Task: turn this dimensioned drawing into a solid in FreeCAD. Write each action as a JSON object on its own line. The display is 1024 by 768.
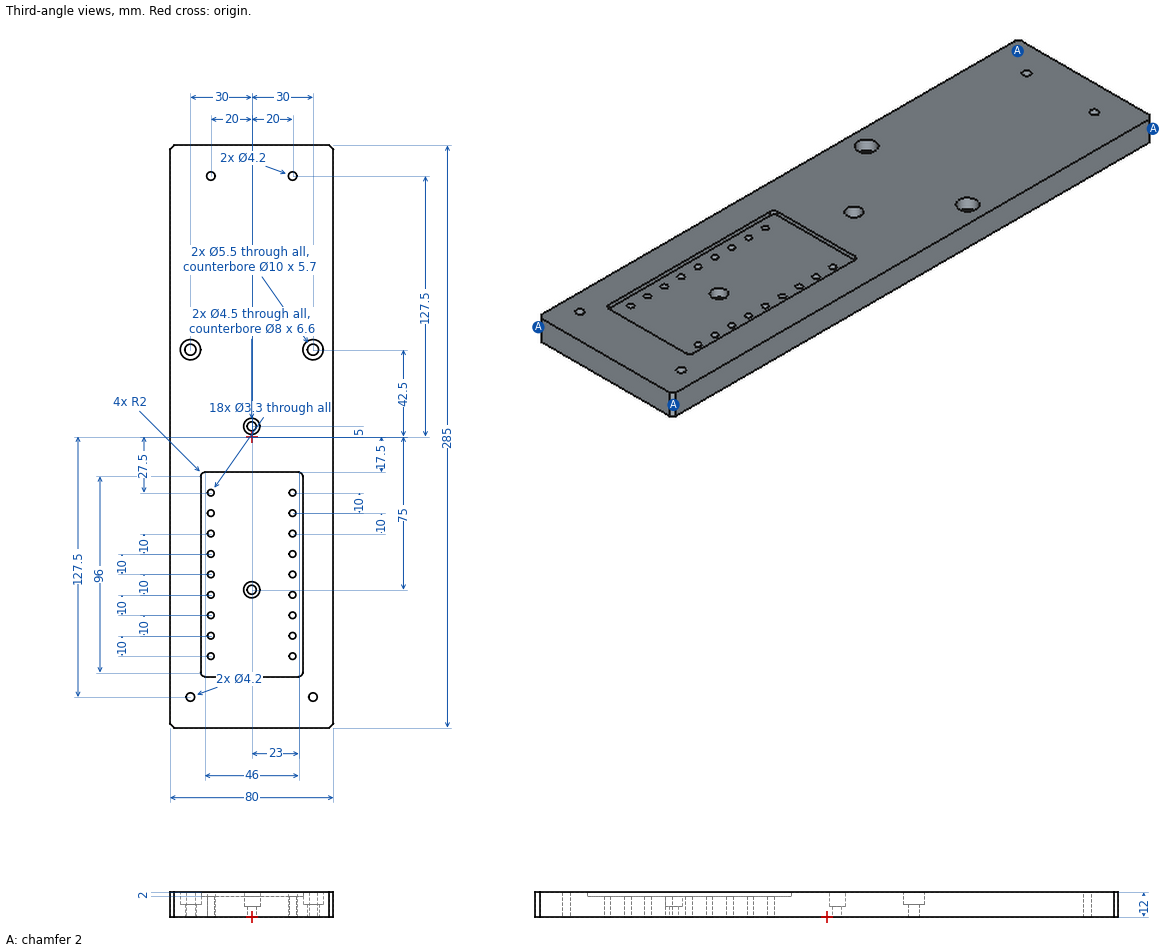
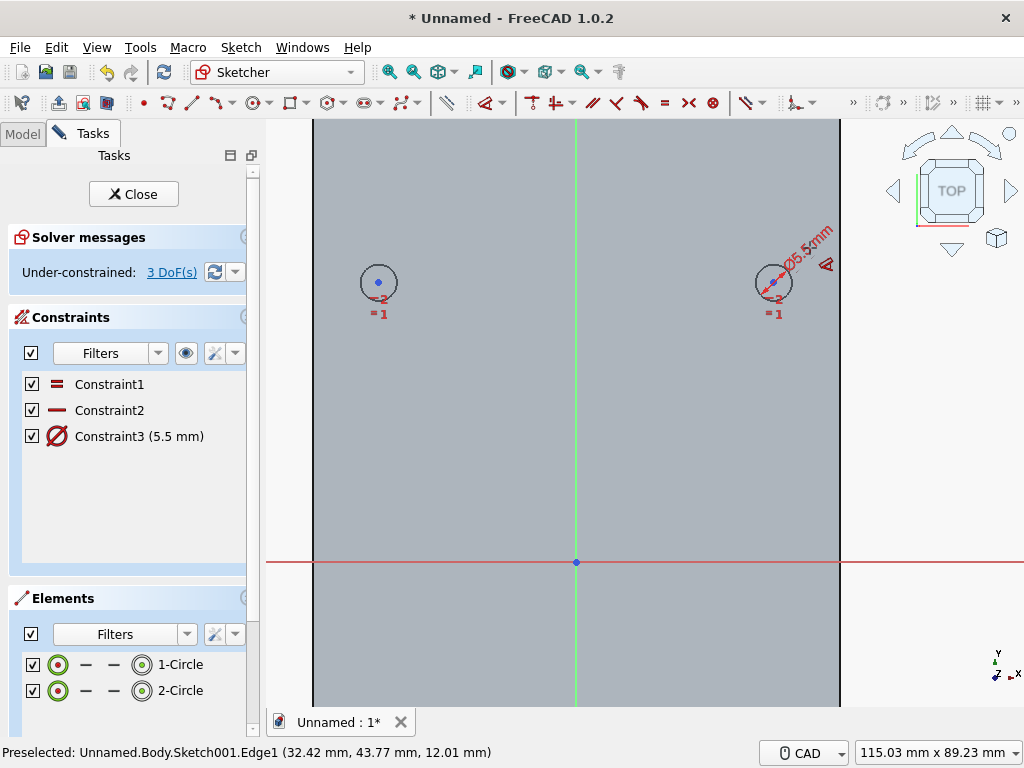
{"action": "left_click", "coordinate": [774, 283]}
{"action": "left_click", "coordinate": [675, 596]}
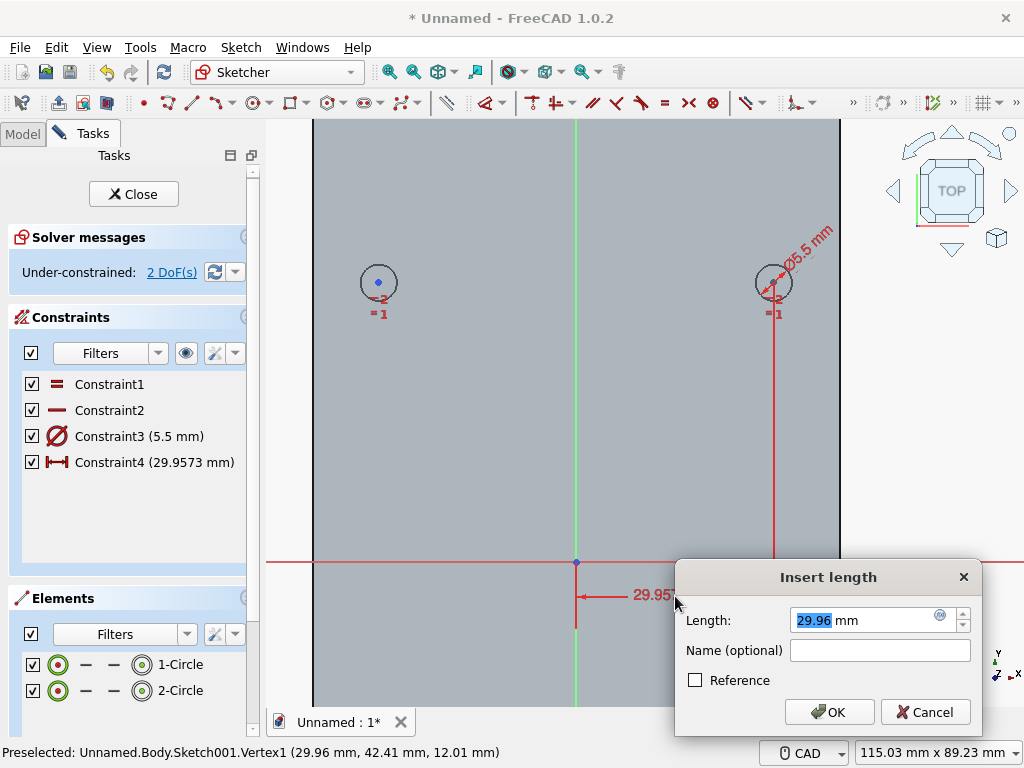
{"action": "type", "text": "30"}
{"action": "key", "text": "Return"}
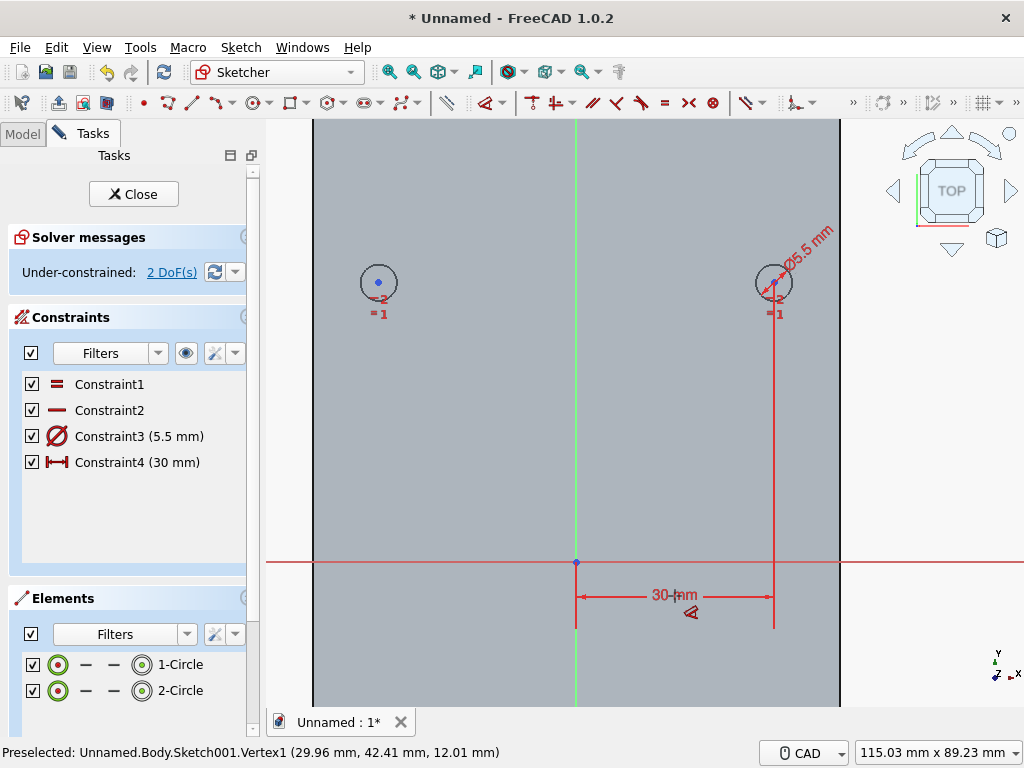
{"action": "left_click", "coordinate": [379, 283]}
{"action": "left_click", "coordinate": [478, 596]}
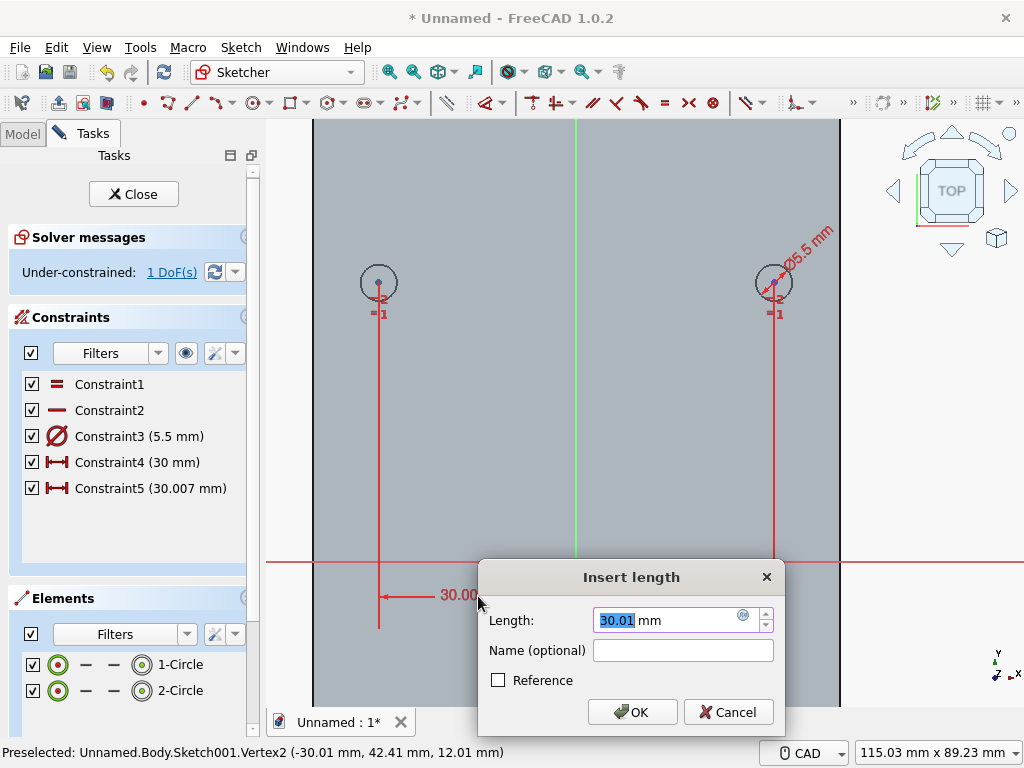
{"action": "type", "text": "30"}
{"action": "key", "text": "Return"}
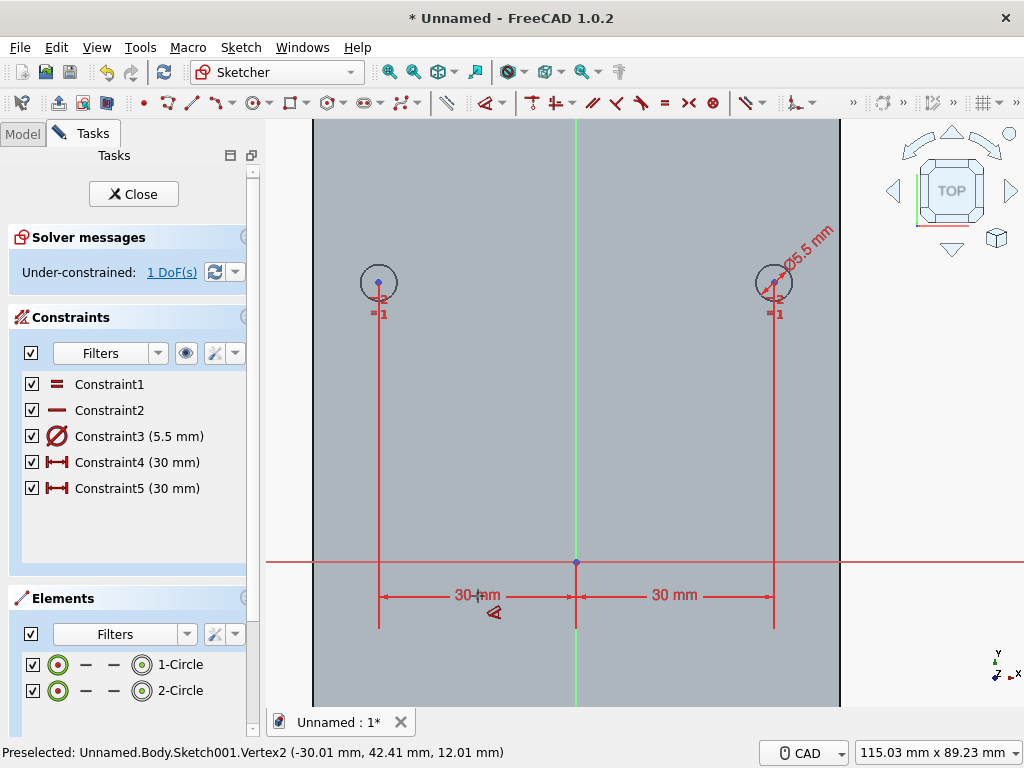
{"action": "left_click", "coordinate": [774, 283]}
{"action": "left_click", "coordinate": [808, 422]}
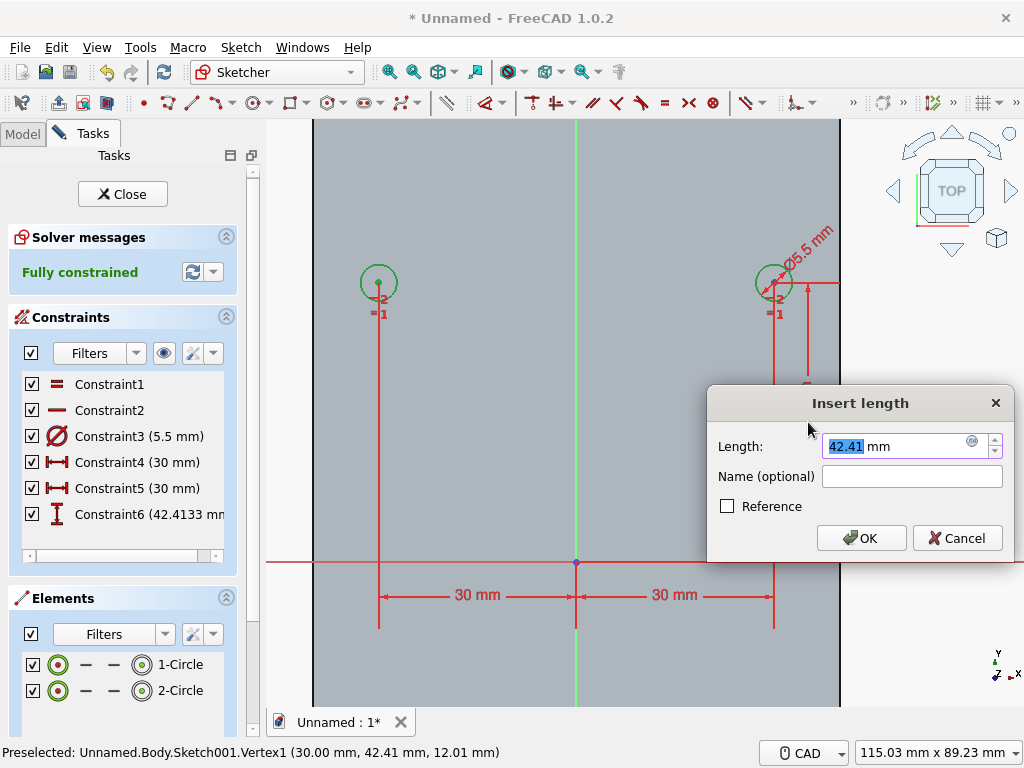
{"action": "type", "text": "42.5"}
{"action": "key", "text": "Return"}
{"action": "key", "text": "Escape"}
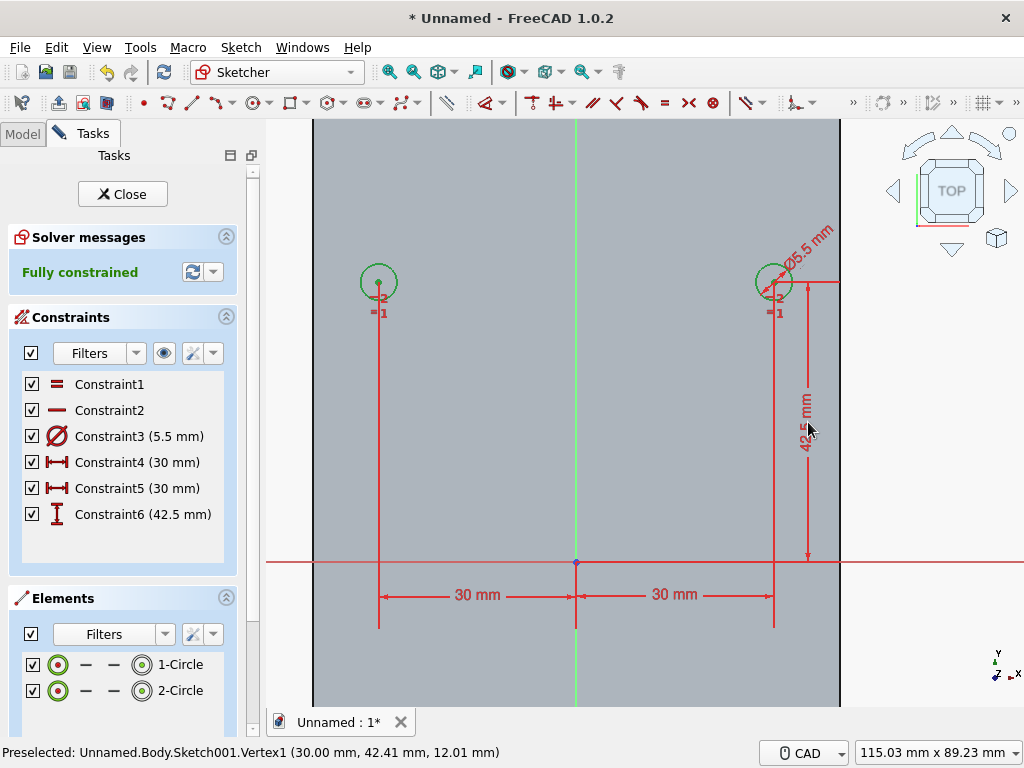
{"action": "left_click", "coordinate": [123, 194]}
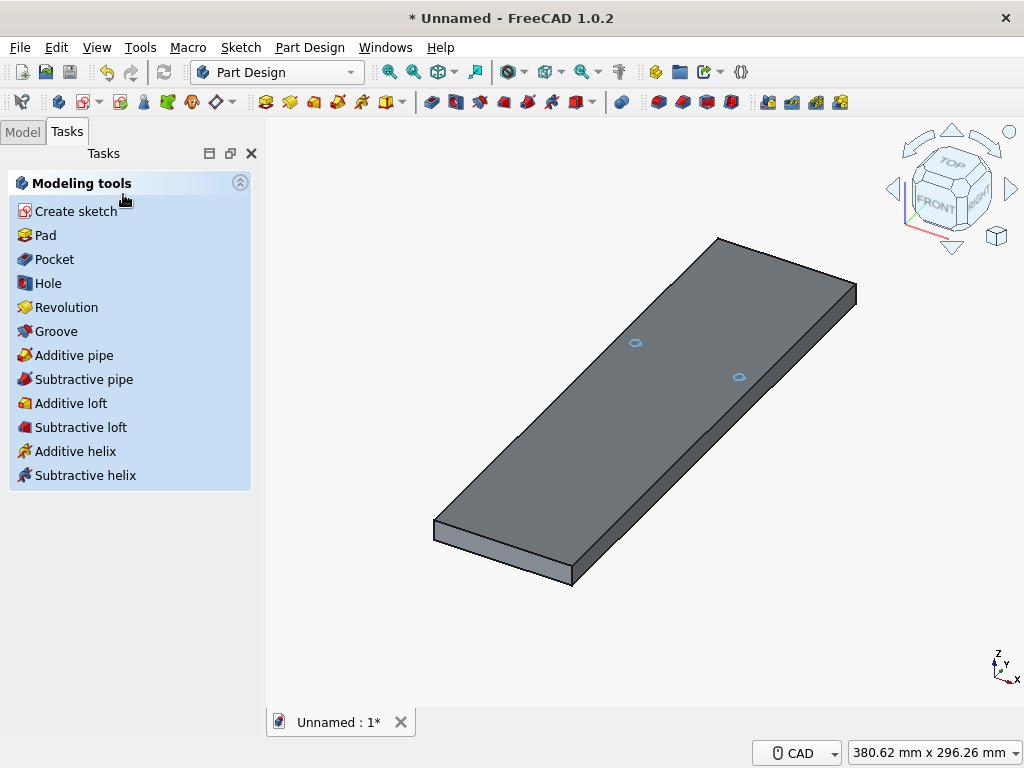
{"action": "left_click", "coordinate": [456, 102]}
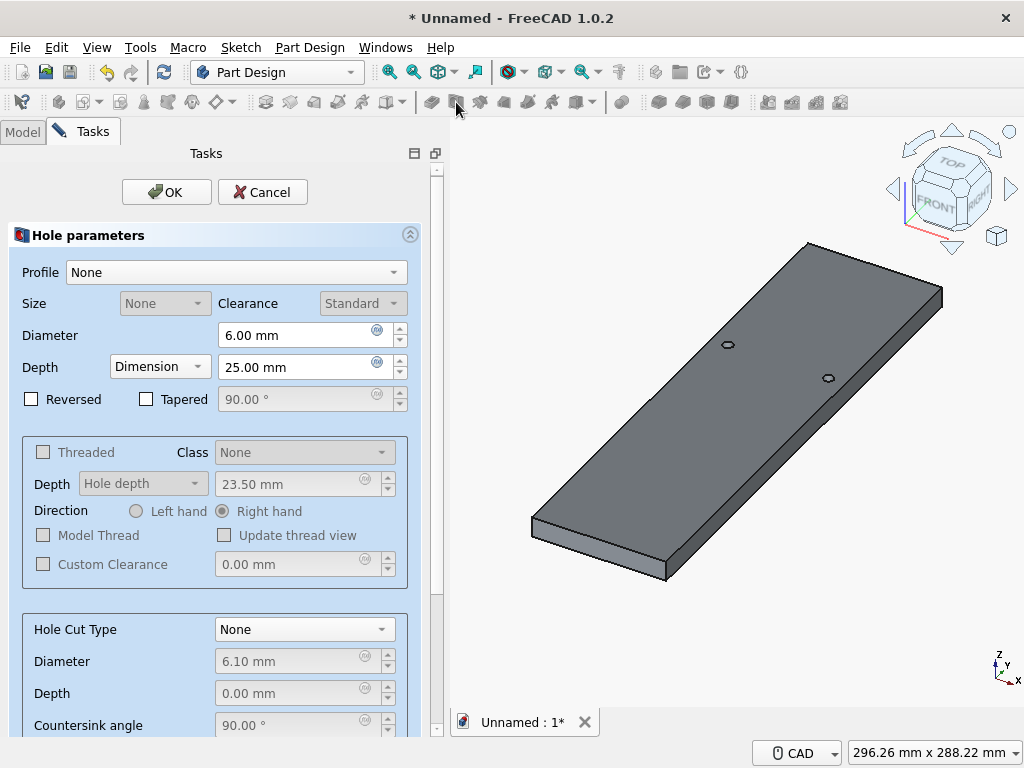
{"action": "triple_click", "coordinate": [305, 335]}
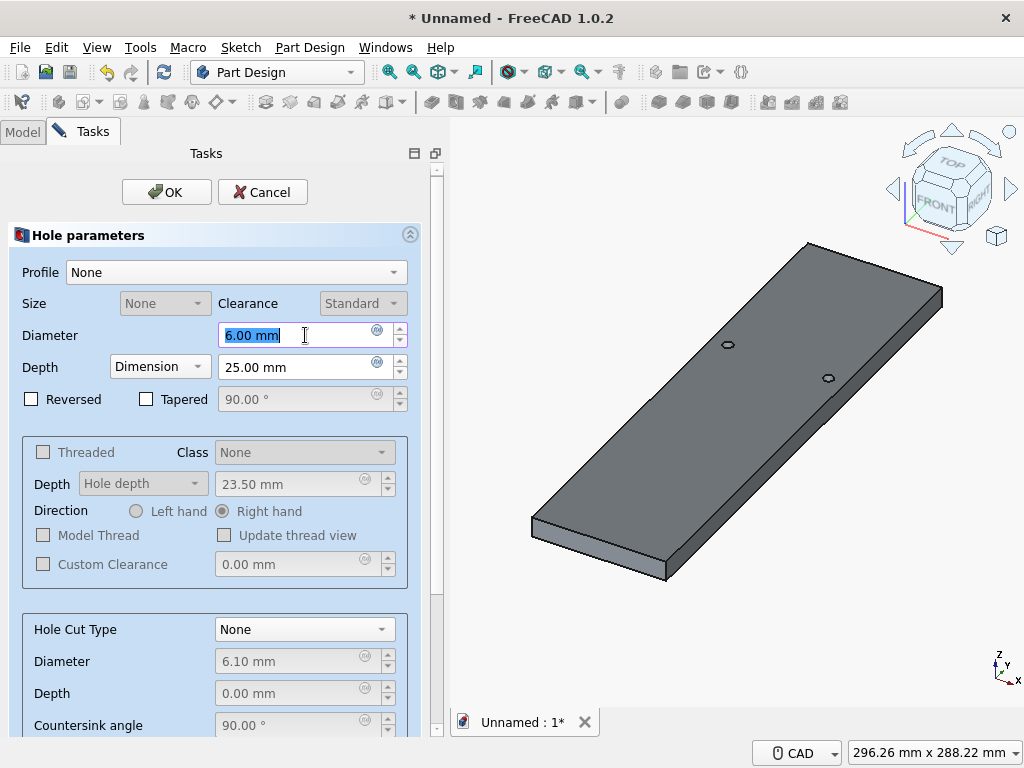
{"action": "type", "text": "5.5"}
{"action": "key", "text": "Tab"}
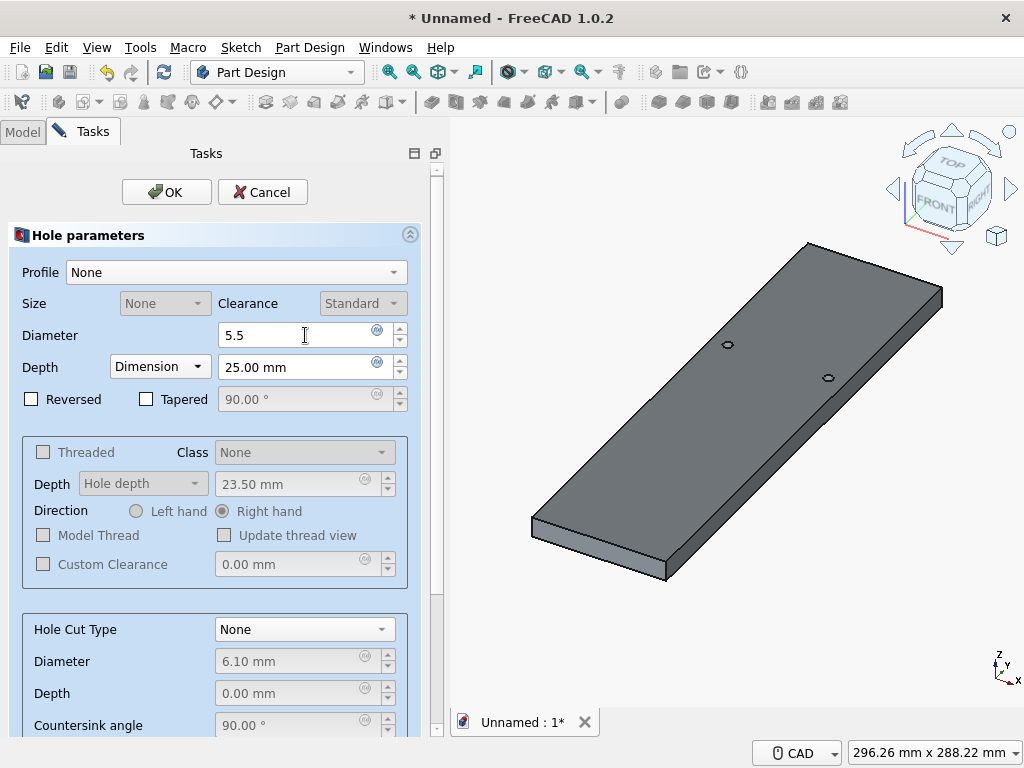
{"action": "left_click", "coordinate": [161, 366]}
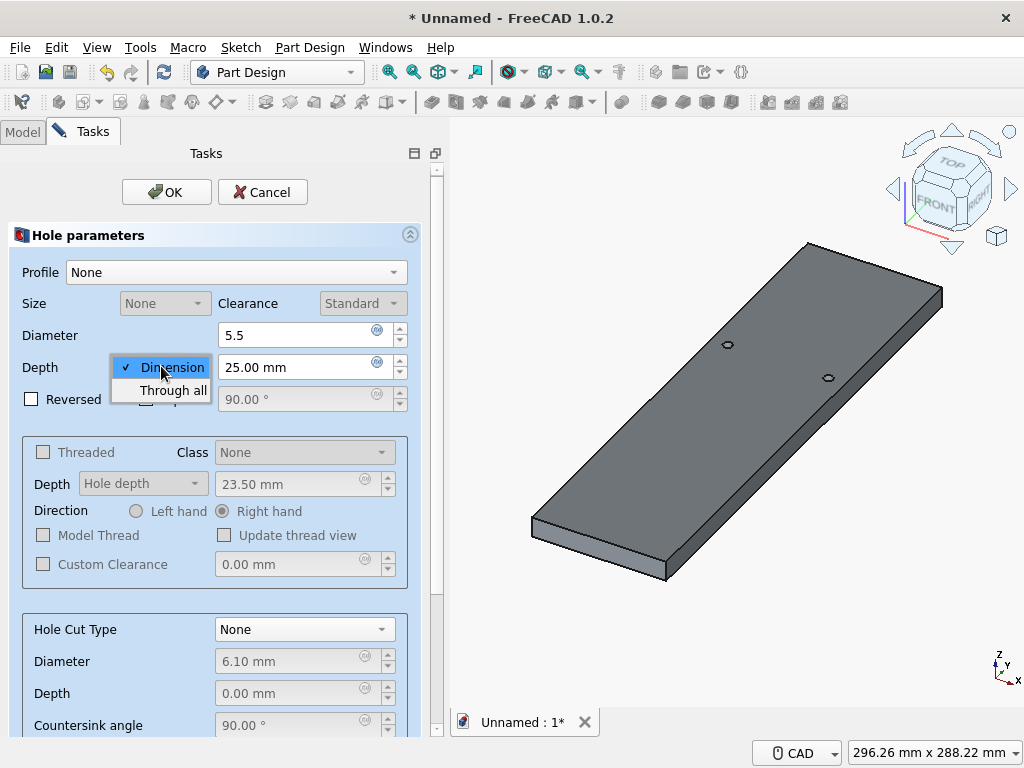
{"action": "left_click", "coordinate": [160, 390]}